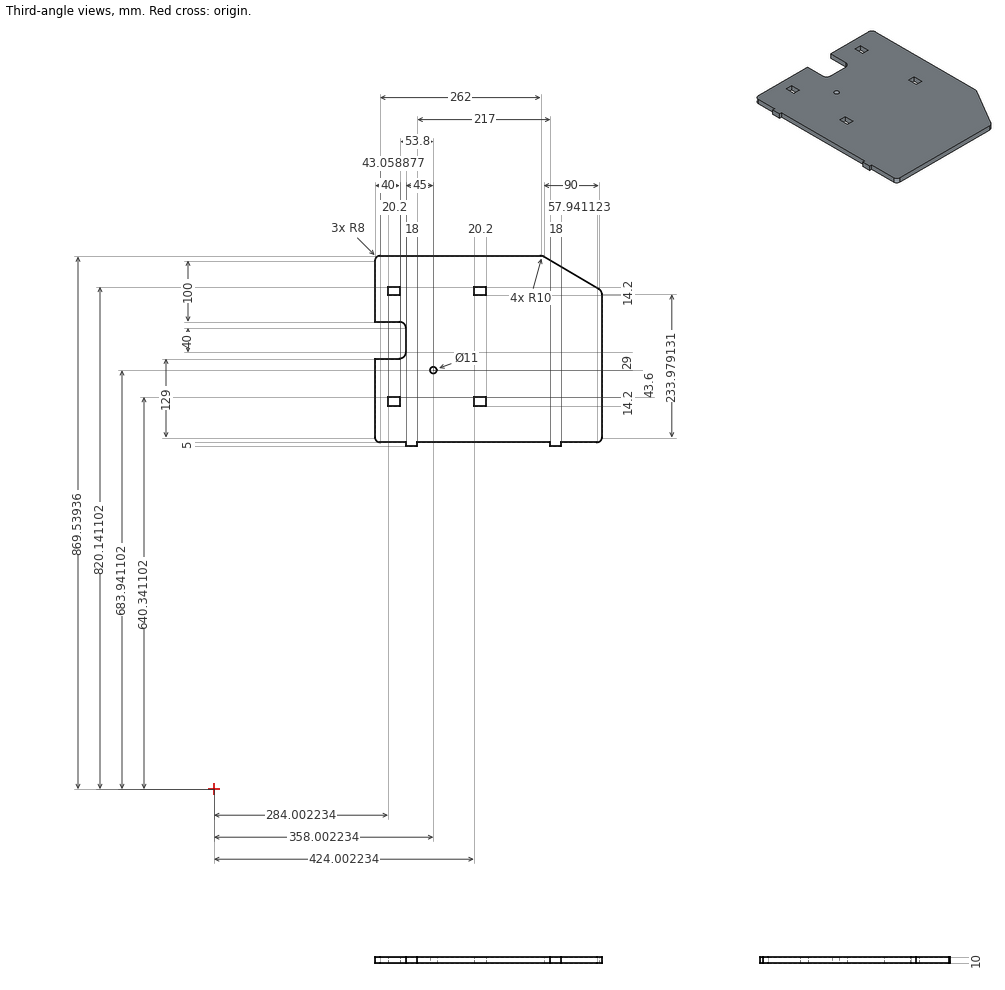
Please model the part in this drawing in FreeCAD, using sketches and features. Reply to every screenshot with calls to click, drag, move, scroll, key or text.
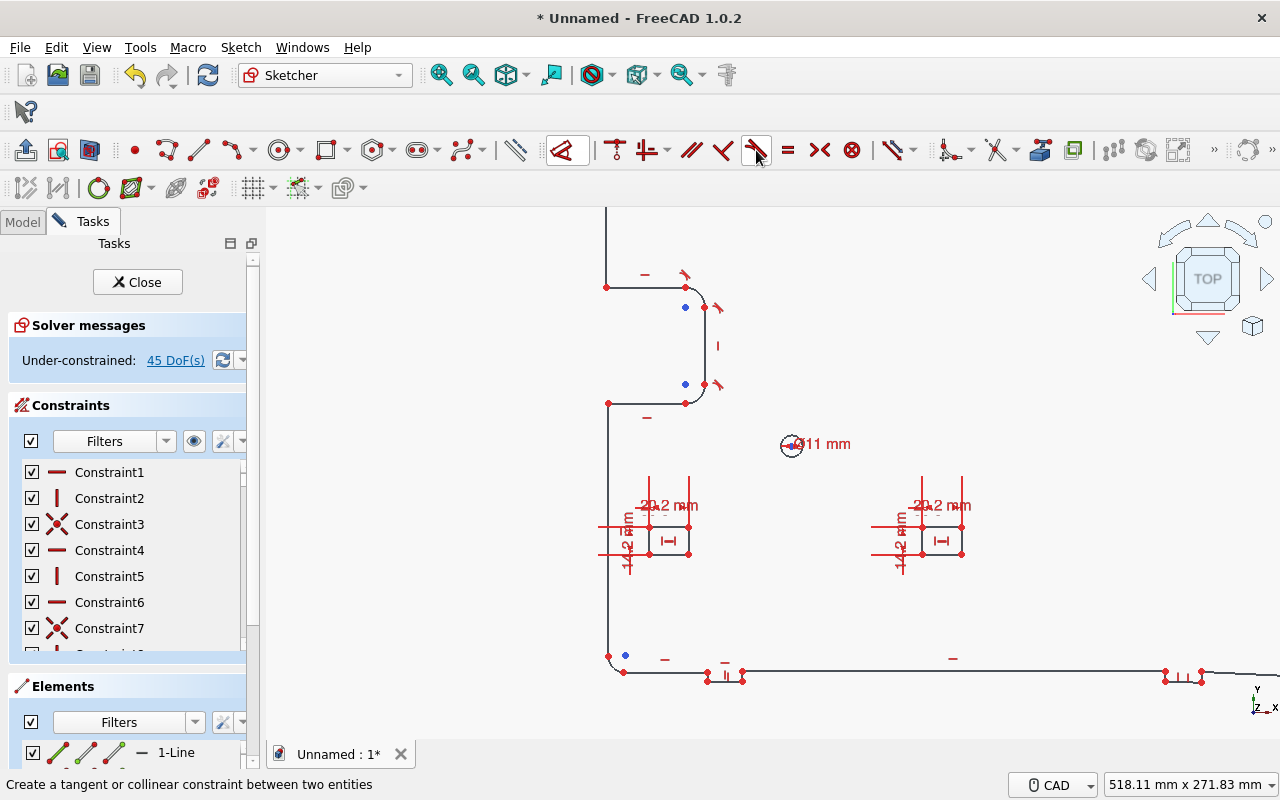
click(662, 404)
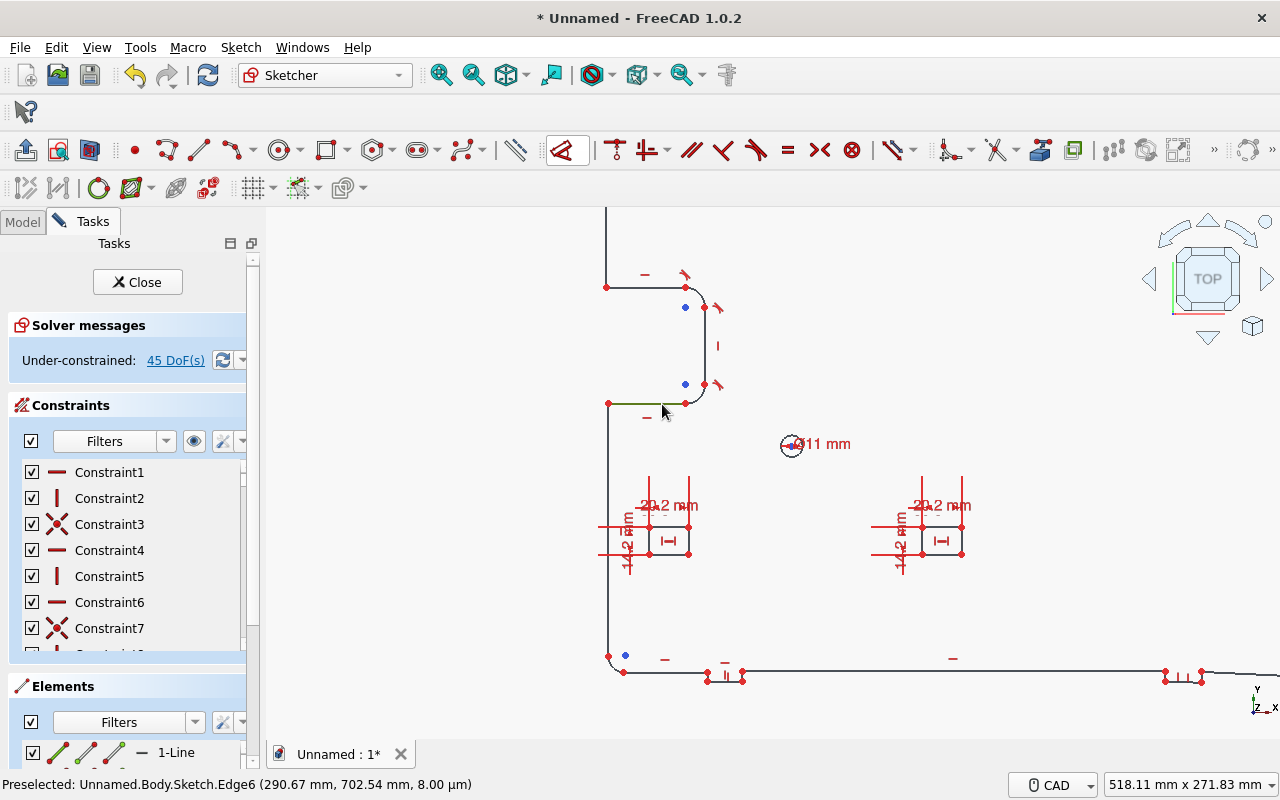
scroll(694, 402, up, 3)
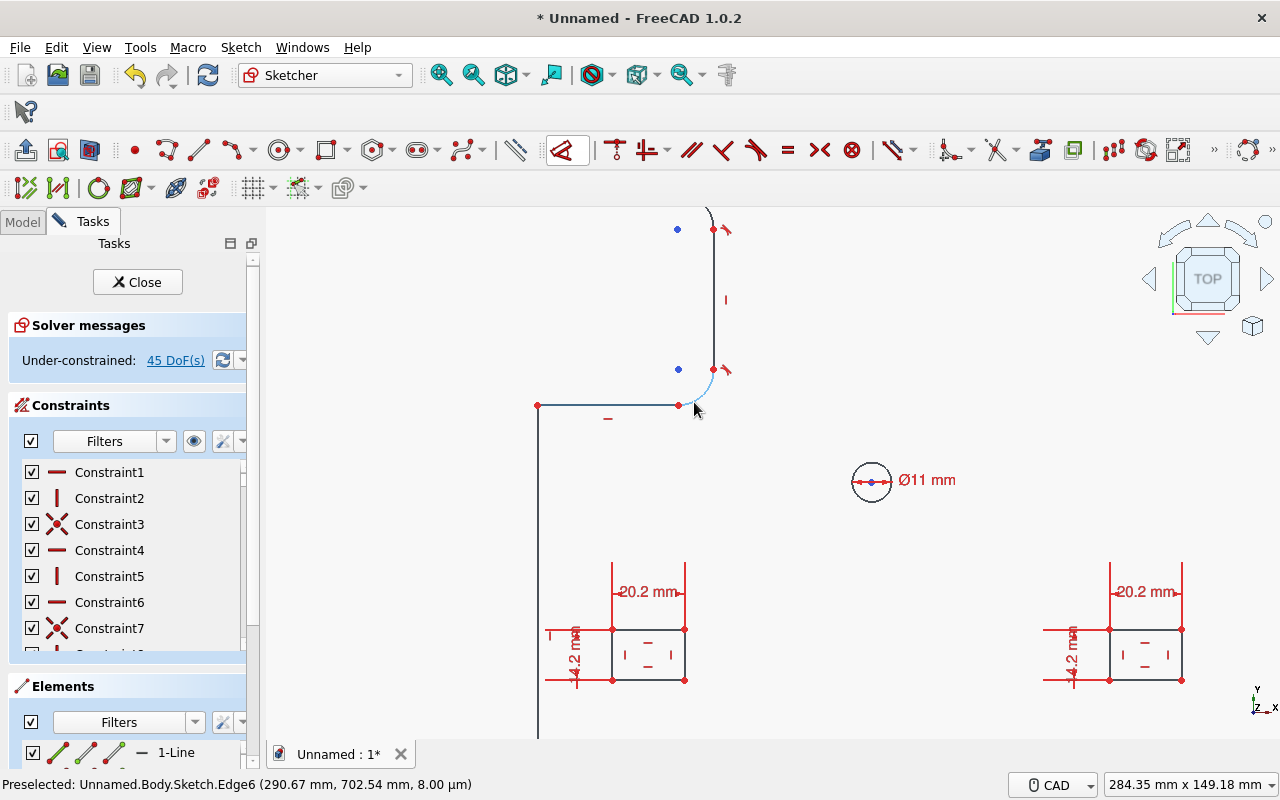
click(694, 401)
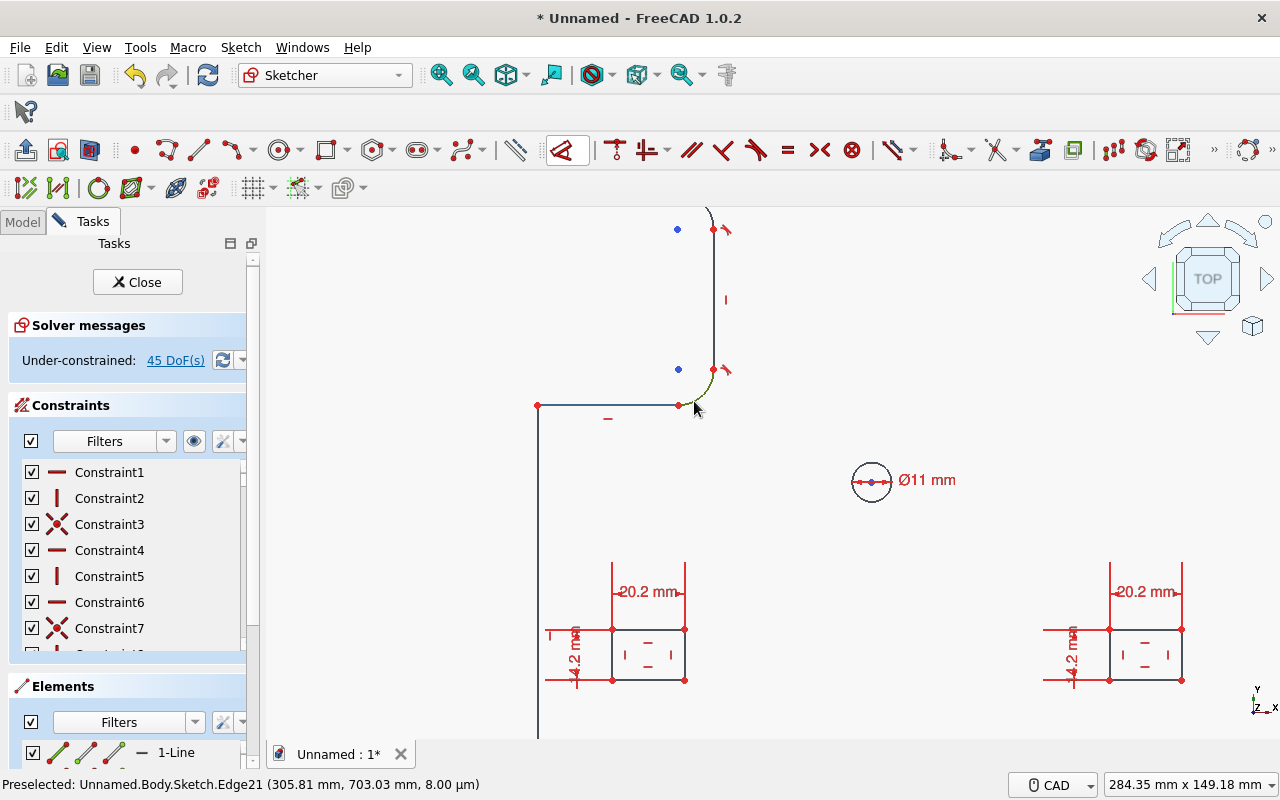
click(756, 150)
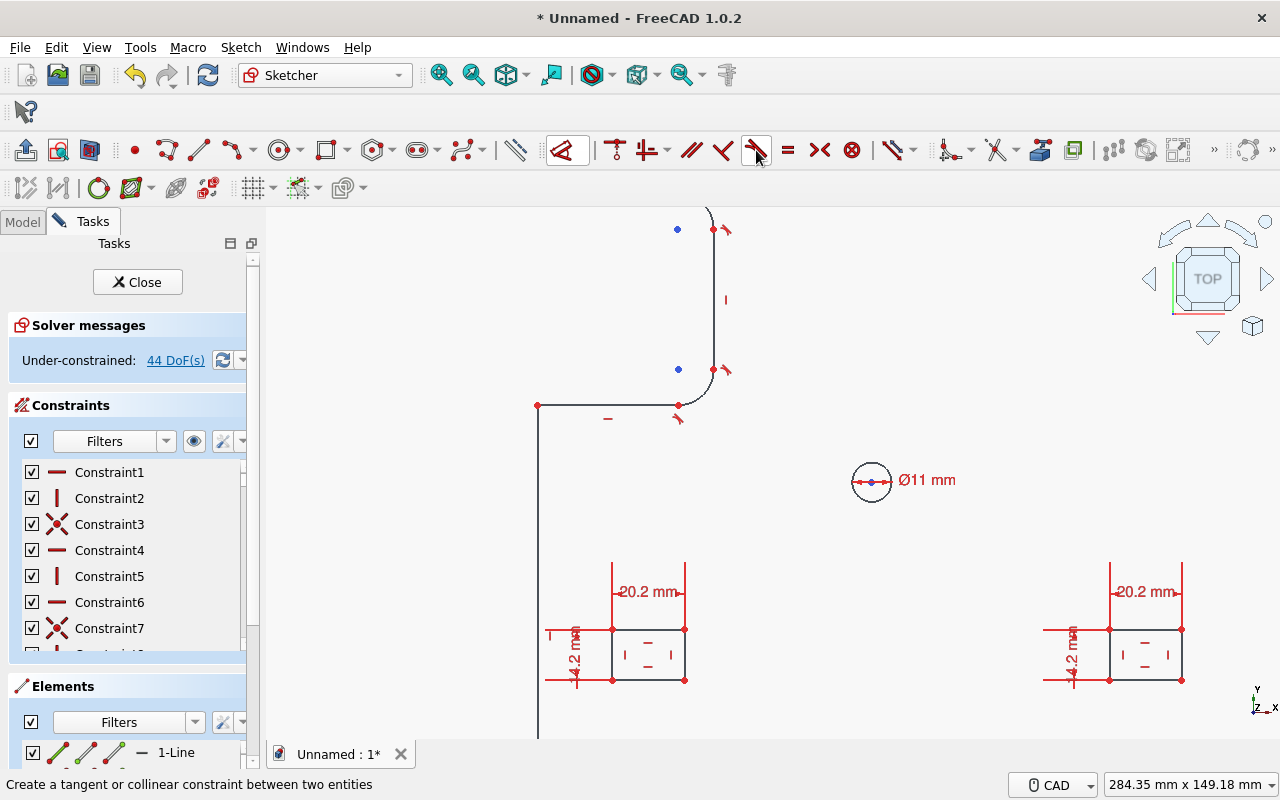
scroll(702, 363, down, 11)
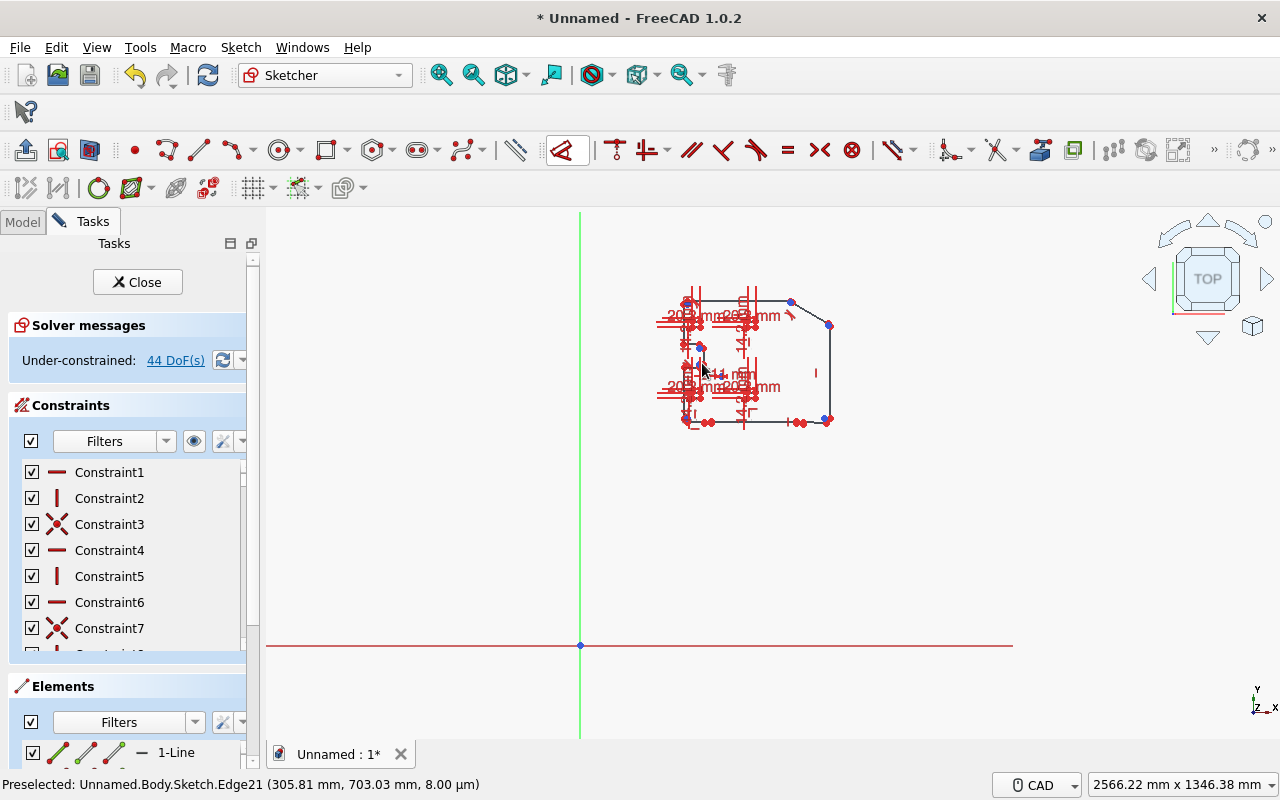
scroll(684, 383, up, 4)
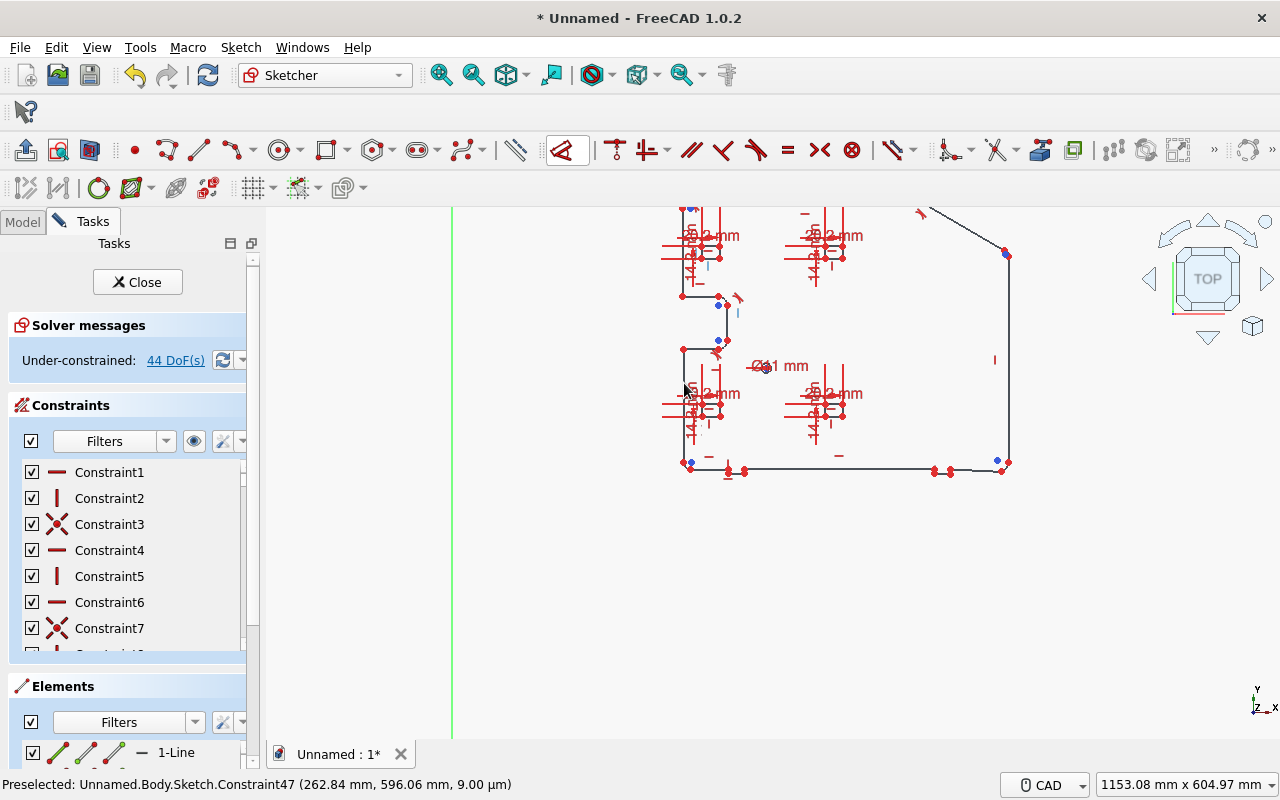
click(684, 383)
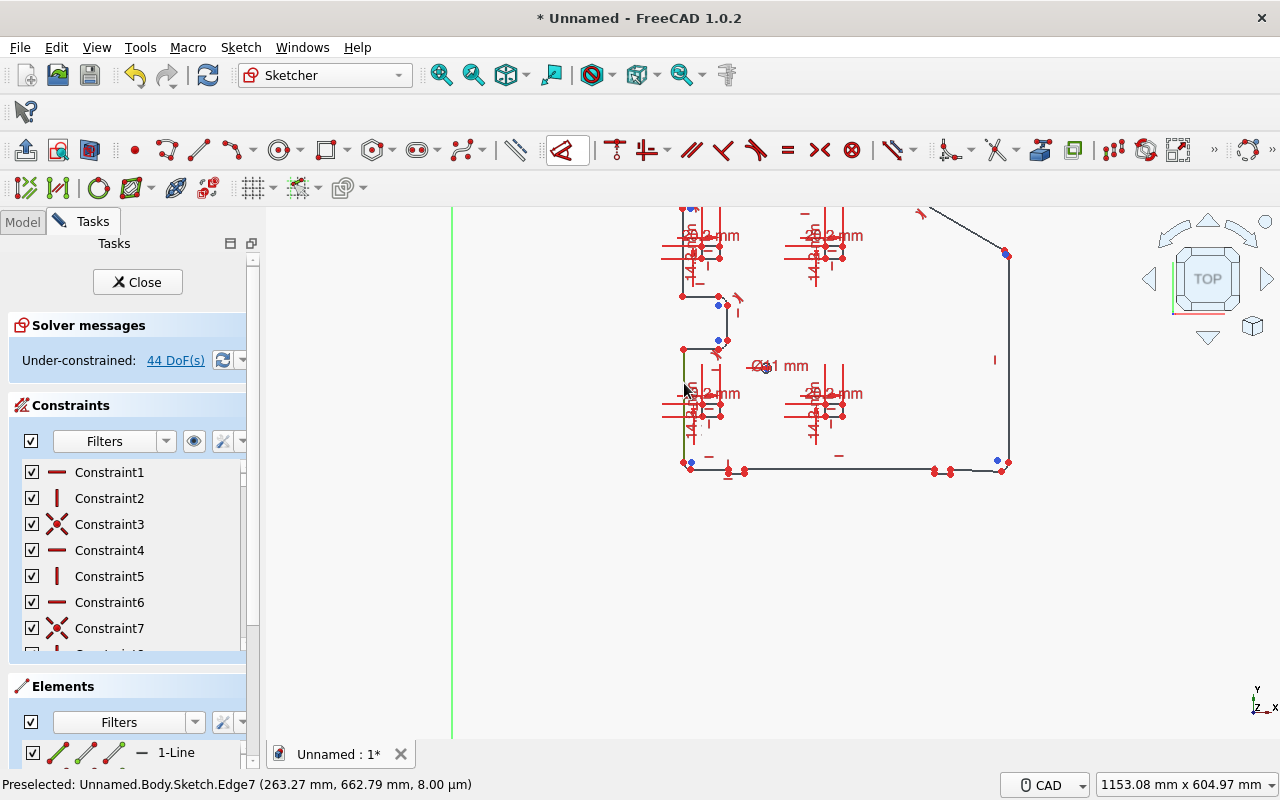
scroll(686, 467, up, 5)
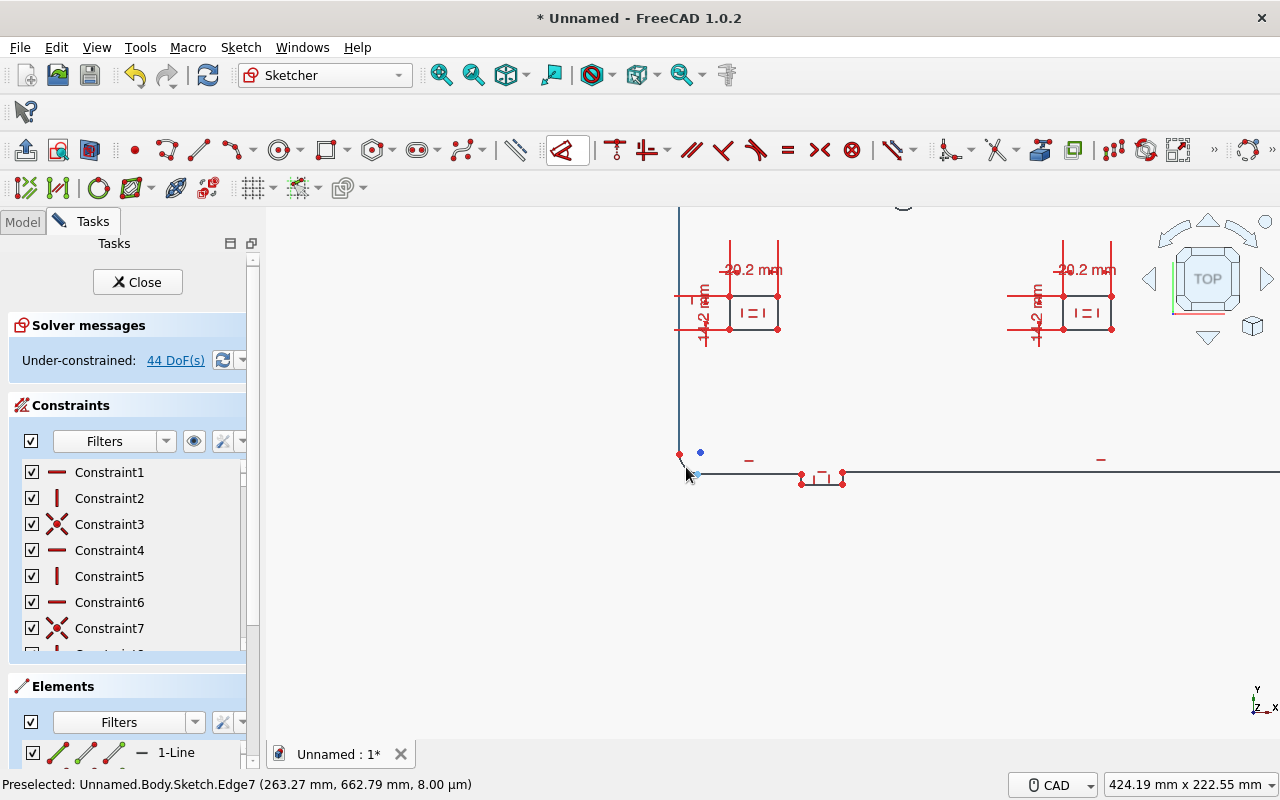
click(685, 467)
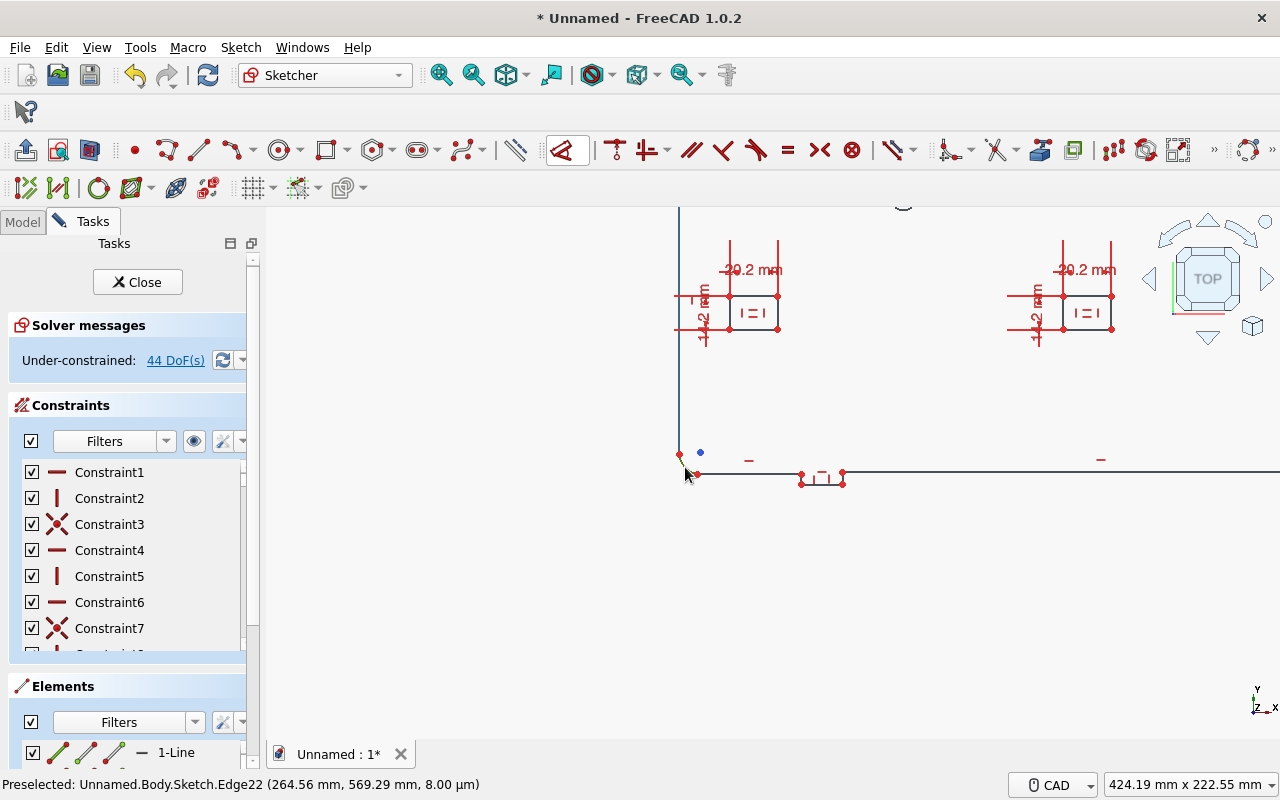
click(756, 150)